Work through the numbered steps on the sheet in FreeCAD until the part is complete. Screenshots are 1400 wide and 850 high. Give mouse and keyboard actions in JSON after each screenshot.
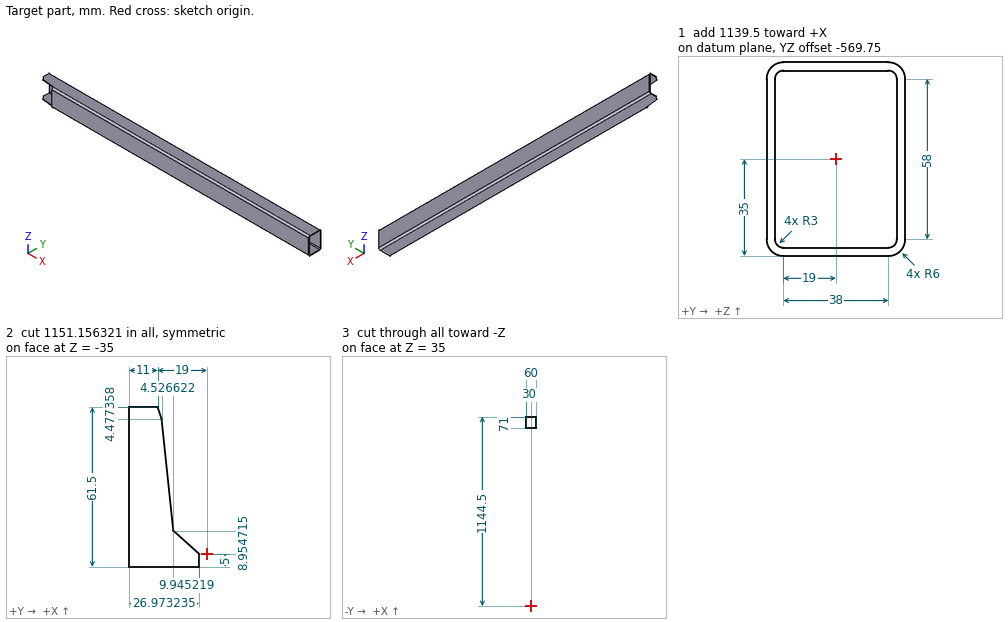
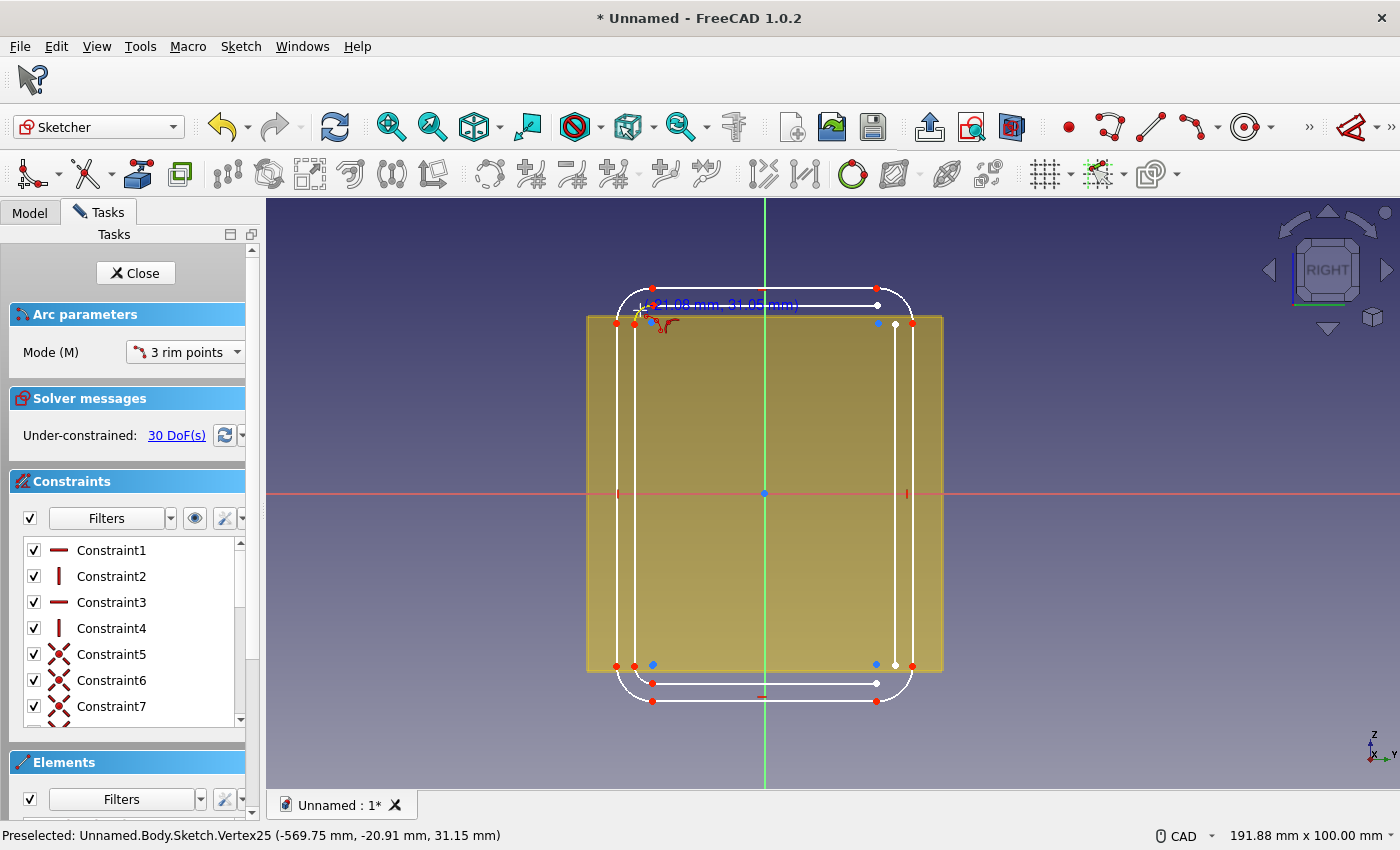
{"action": "left_click", "coordinate": [877, 306]}
{"action": "left_click", "coordinate": [895, 324]}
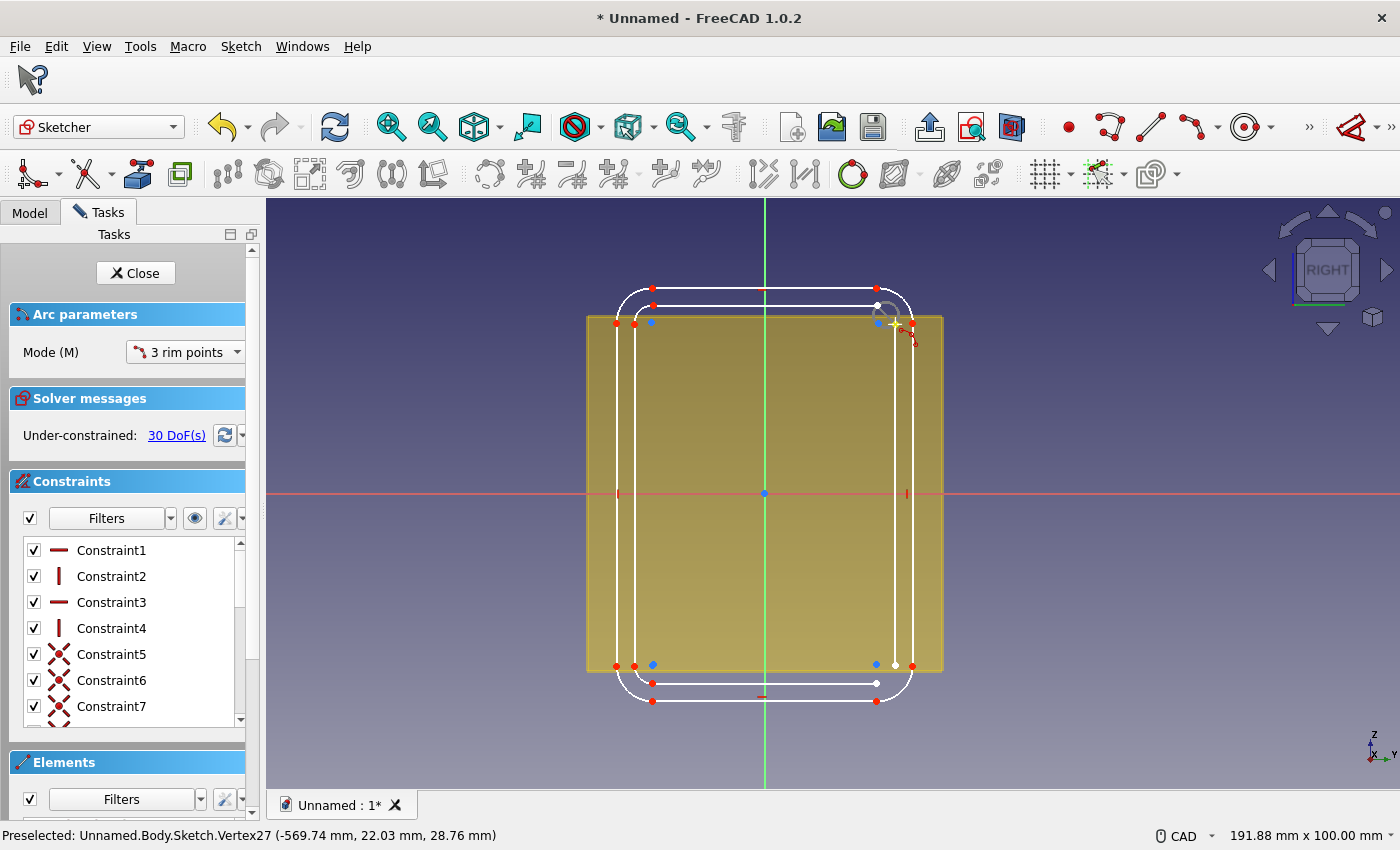
{"action": "scroll", "coordinate": [890, 310], "scroll_direction": "up", "scroll_amount": 6}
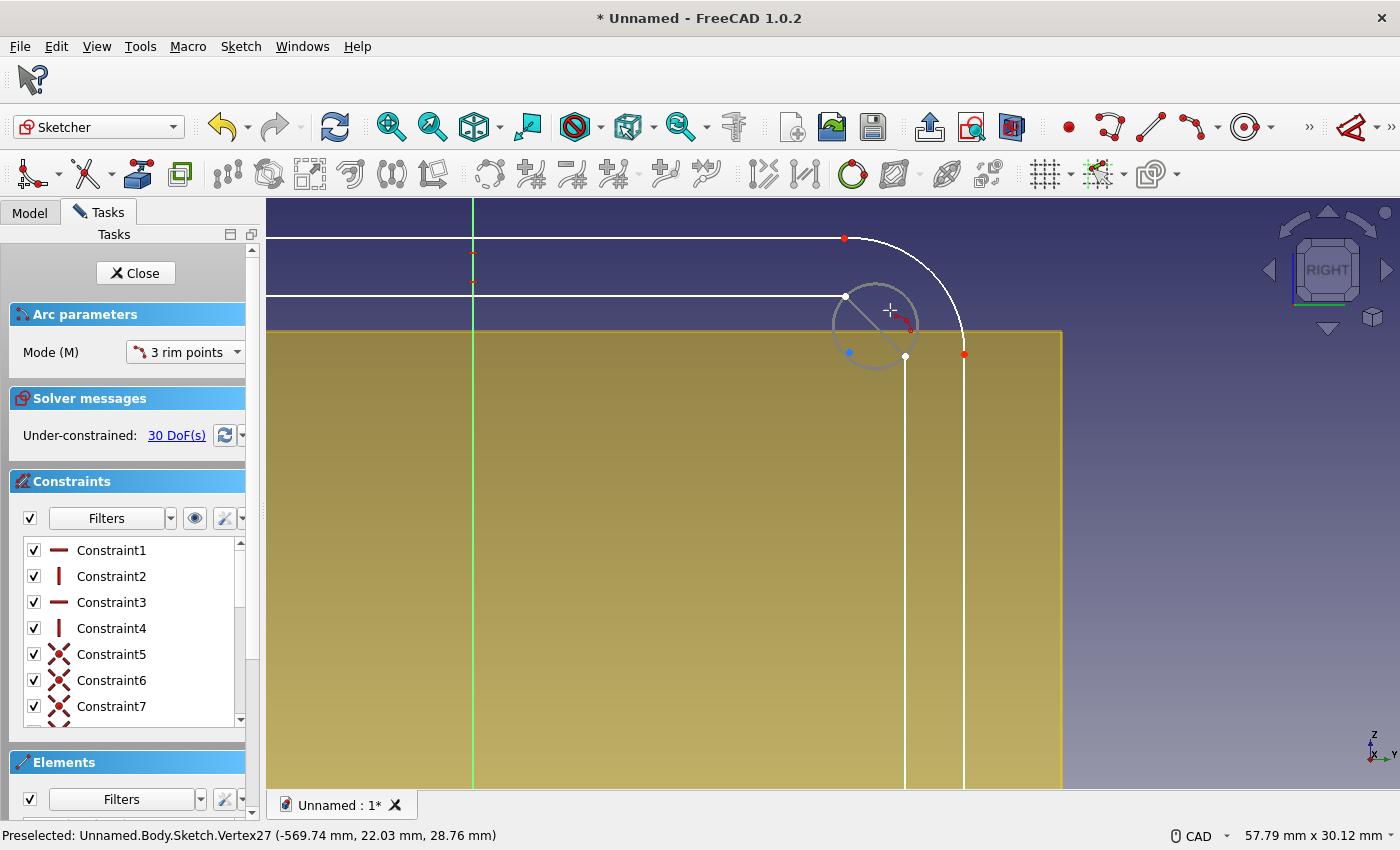
{"action": "left_click", "coordinate": [888, 310]}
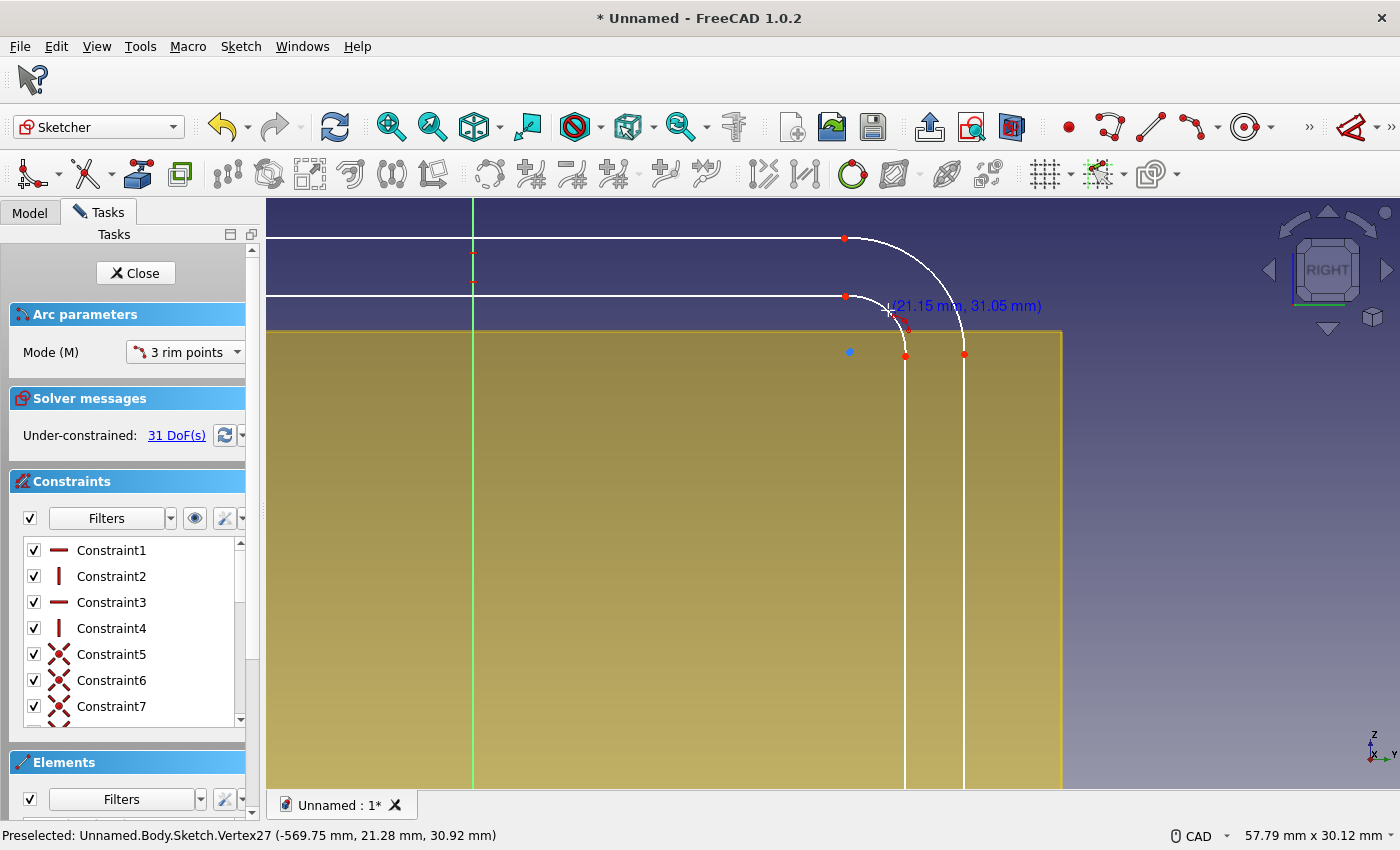
{"action": "scroll", "coordinate": [890, 310], "scroll_direction": "down", "scroll_amount": 6}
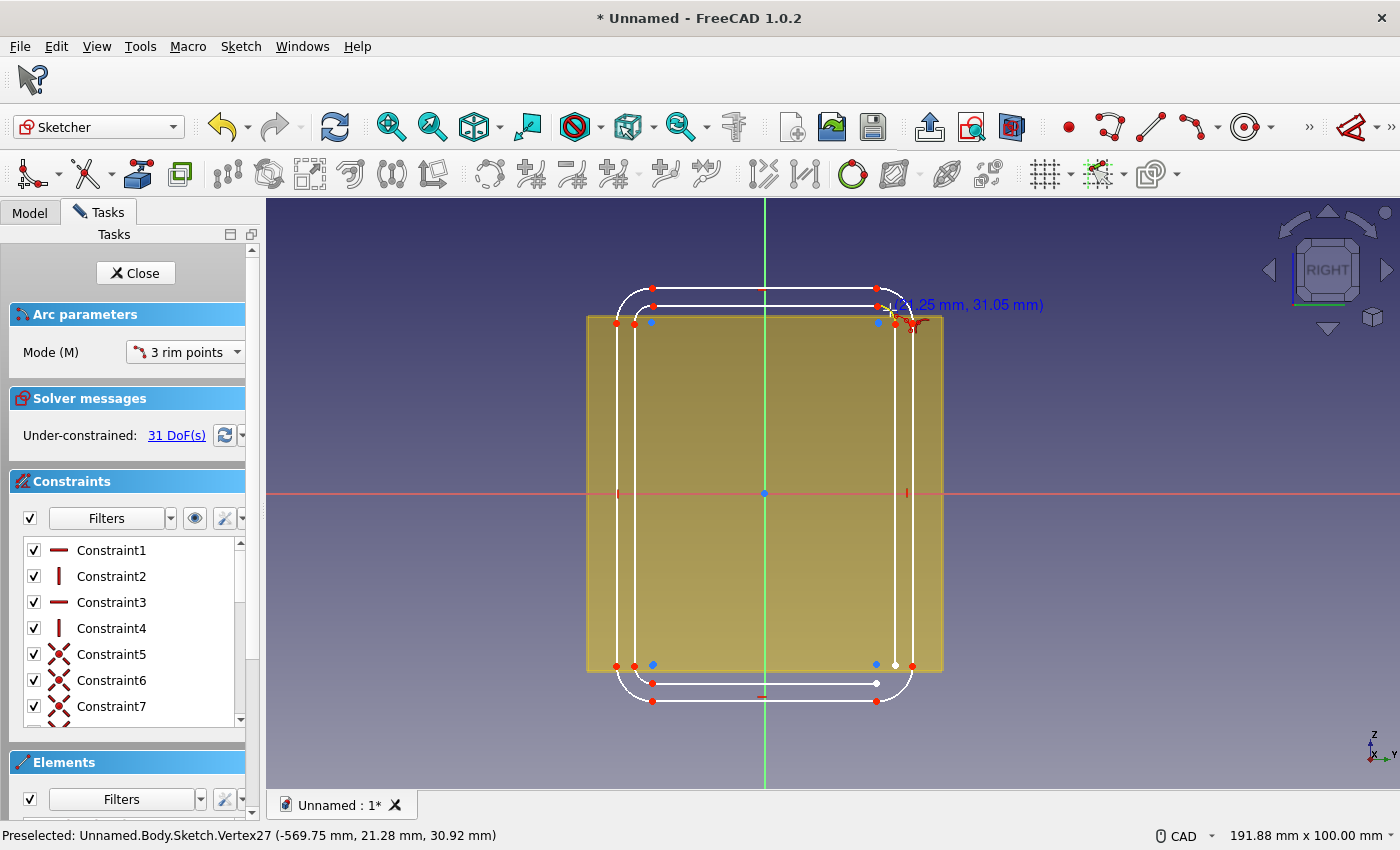
{"action": "left_click", "coordinate": [895, 666]}
{"action": "left_click", "coordinate": [877, 684]}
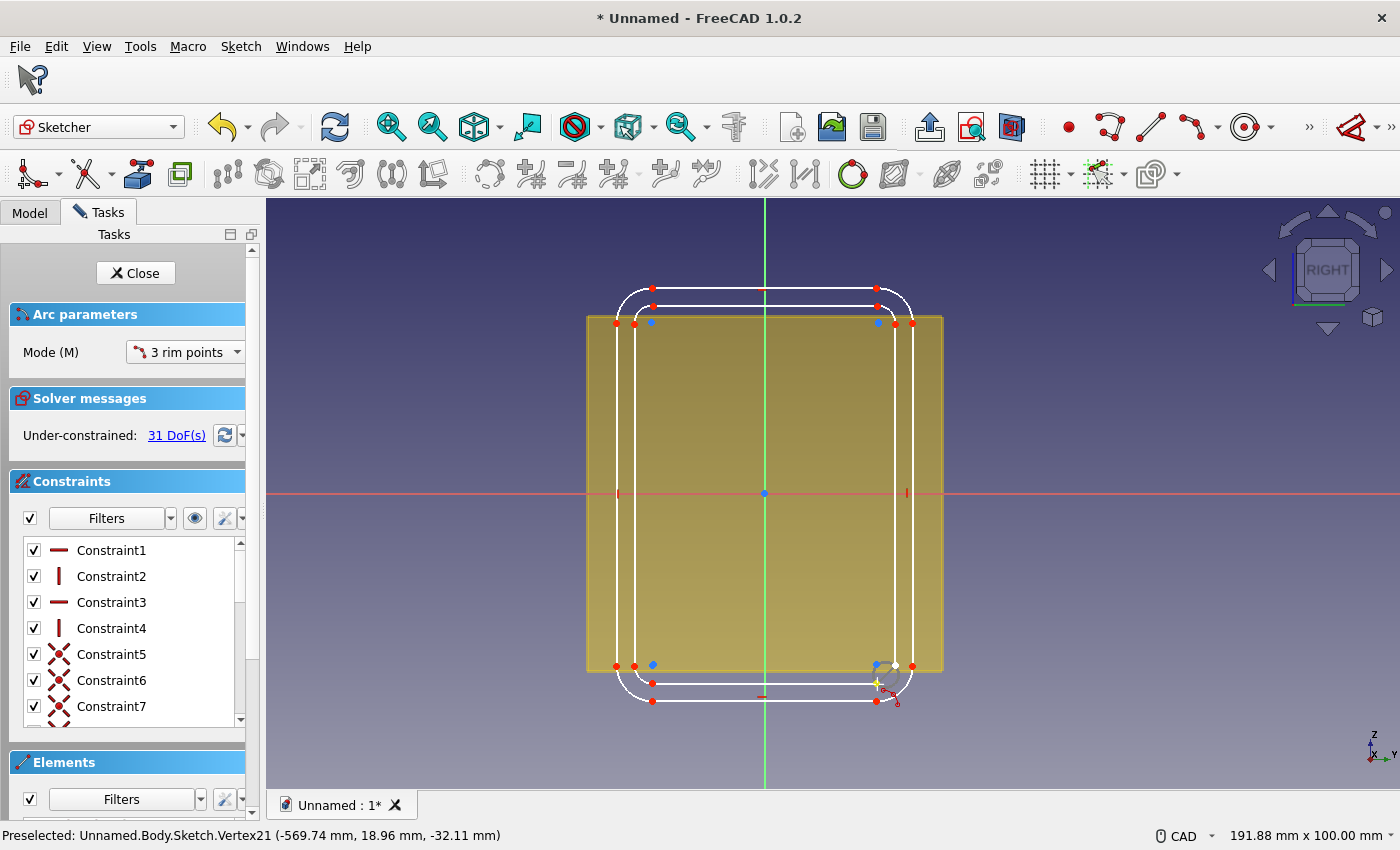
{"action": "scroll", "coordinate": [890, 678], "scroll_direction": "up", "scroll_amount": 6}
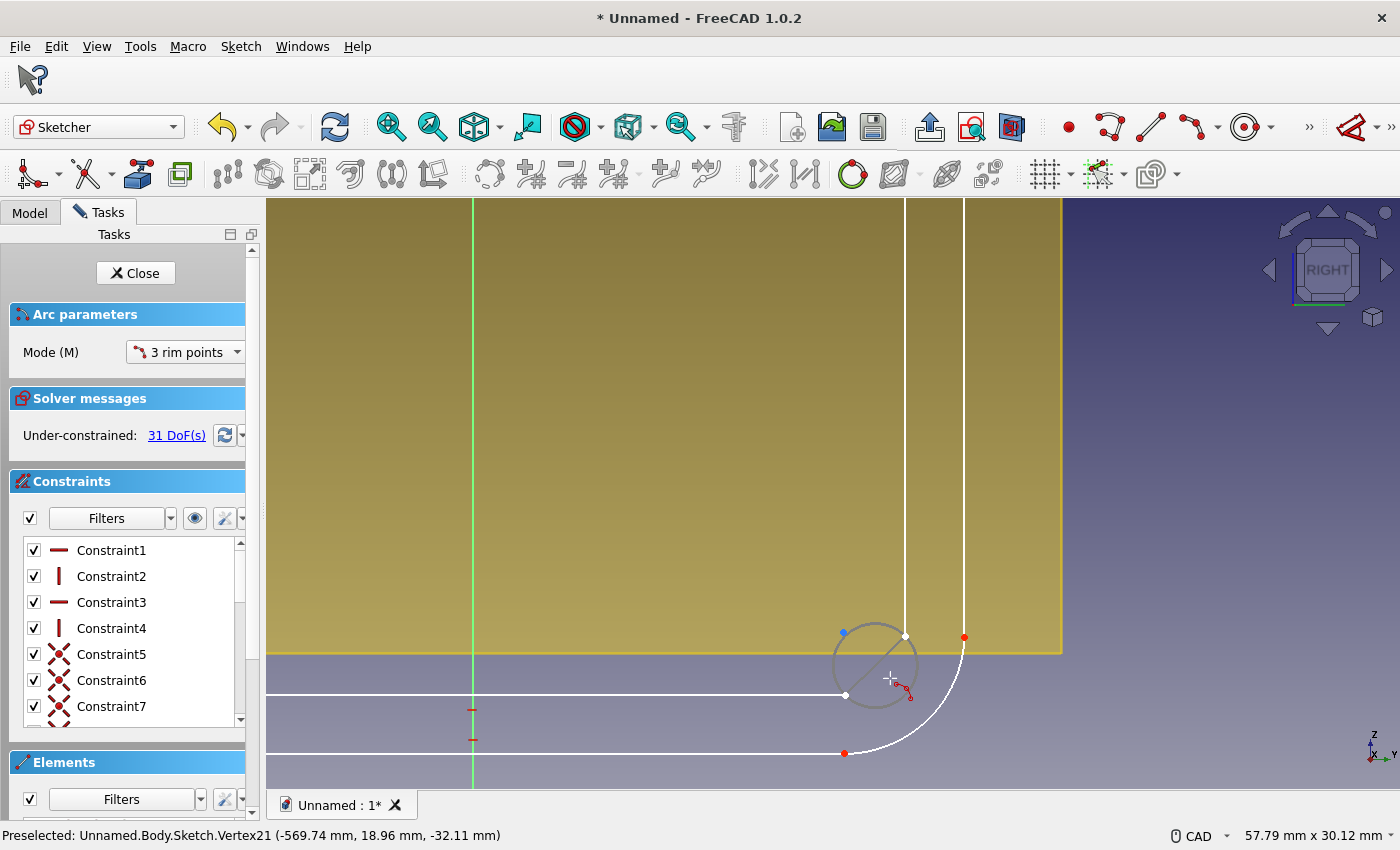
{"action": "left_click", "coordinate": [888, 676]}
{"action": "key", "text": "Escape"}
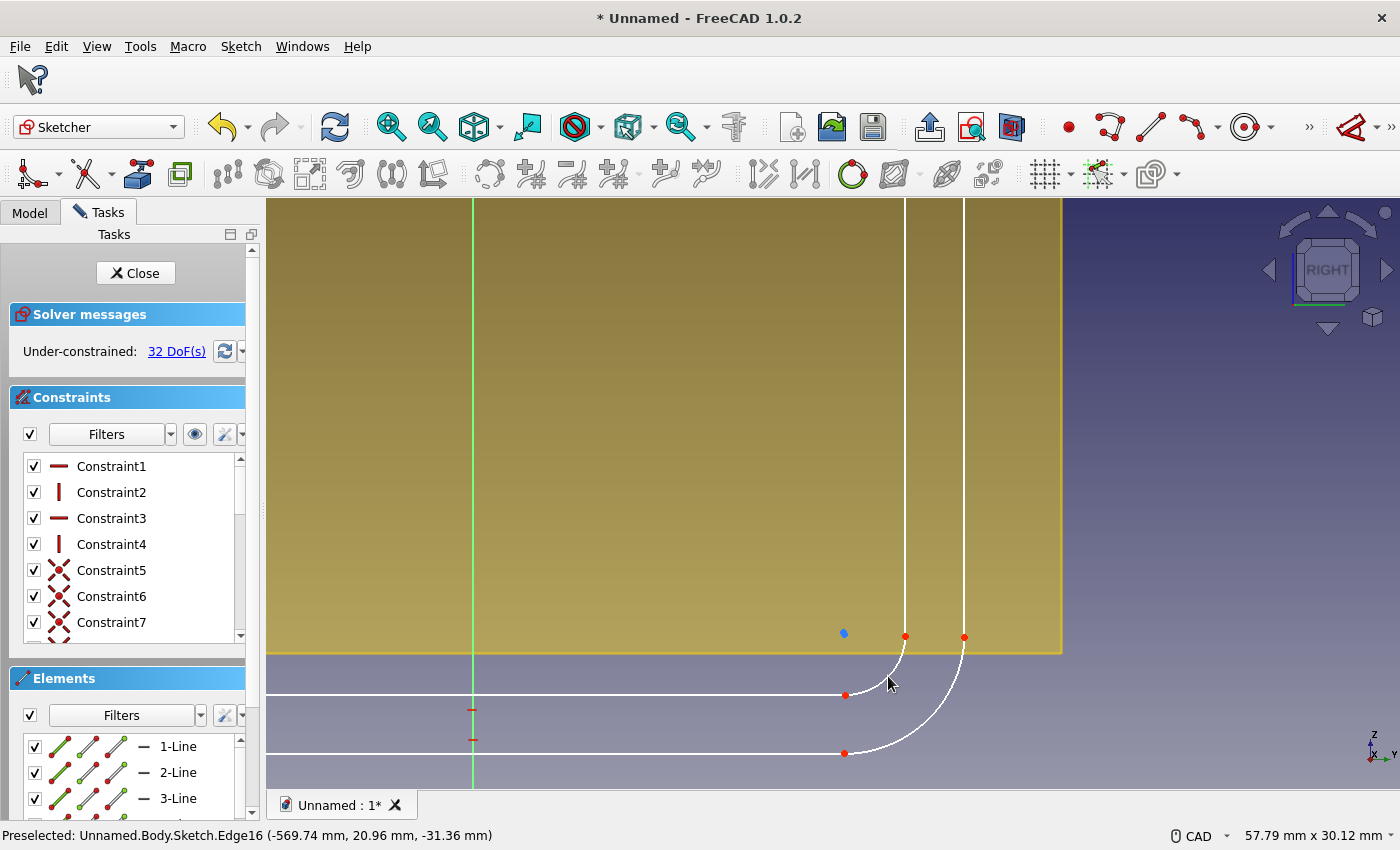
{"action": "left_click", "coordinate": [324, 754]}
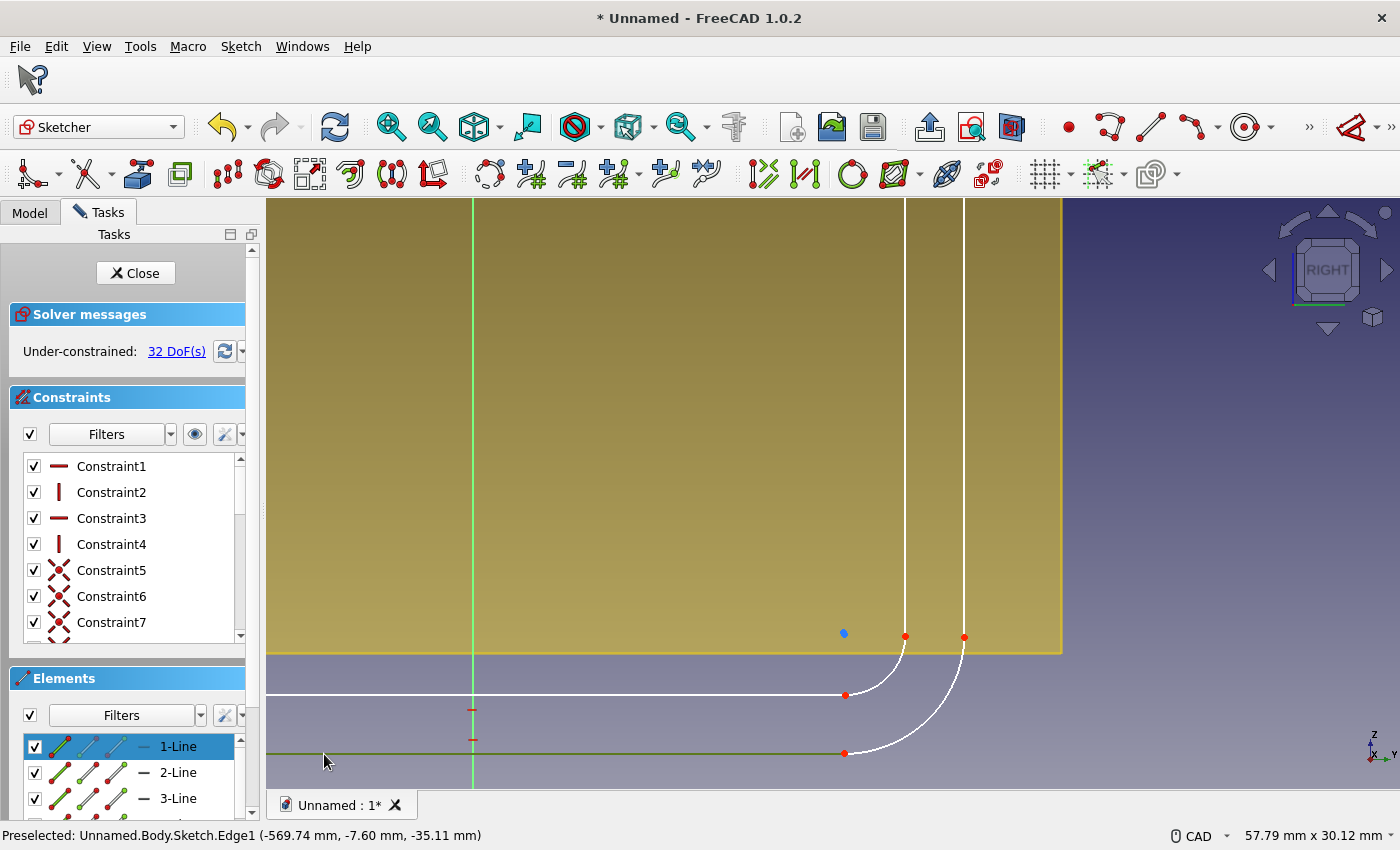
{"action": "left_click", "coordinate": [898, 741]}